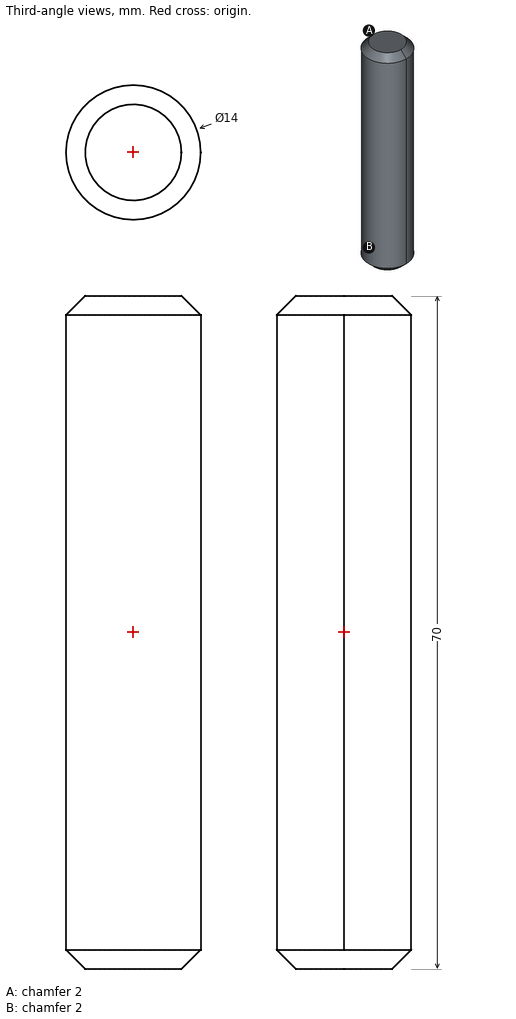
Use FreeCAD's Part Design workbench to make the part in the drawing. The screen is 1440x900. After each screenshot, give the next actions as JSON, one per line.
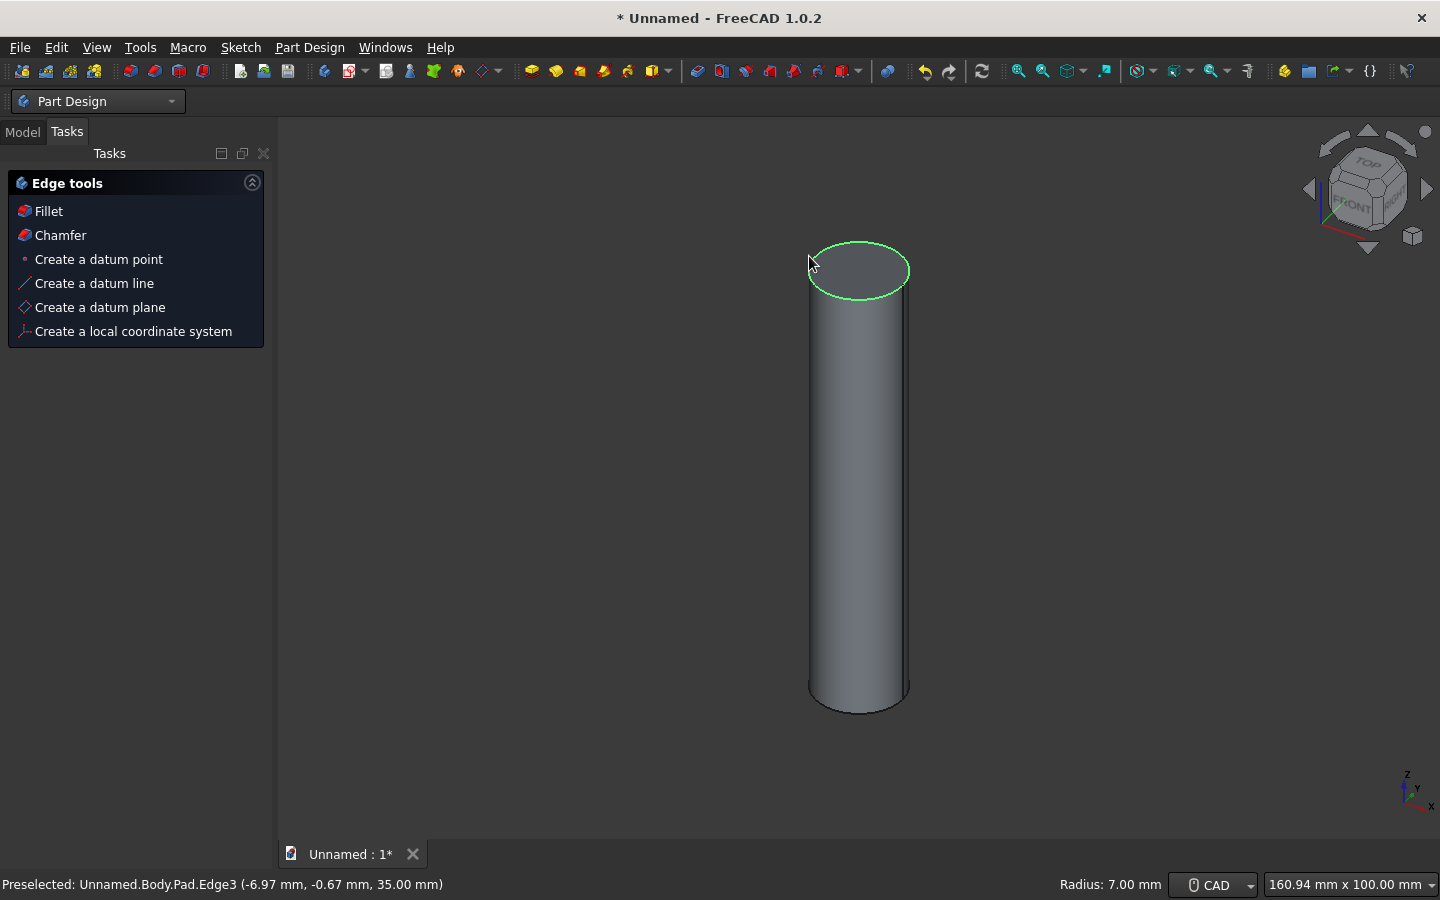
{"action": "left_click", "coordinate": [156, 72]}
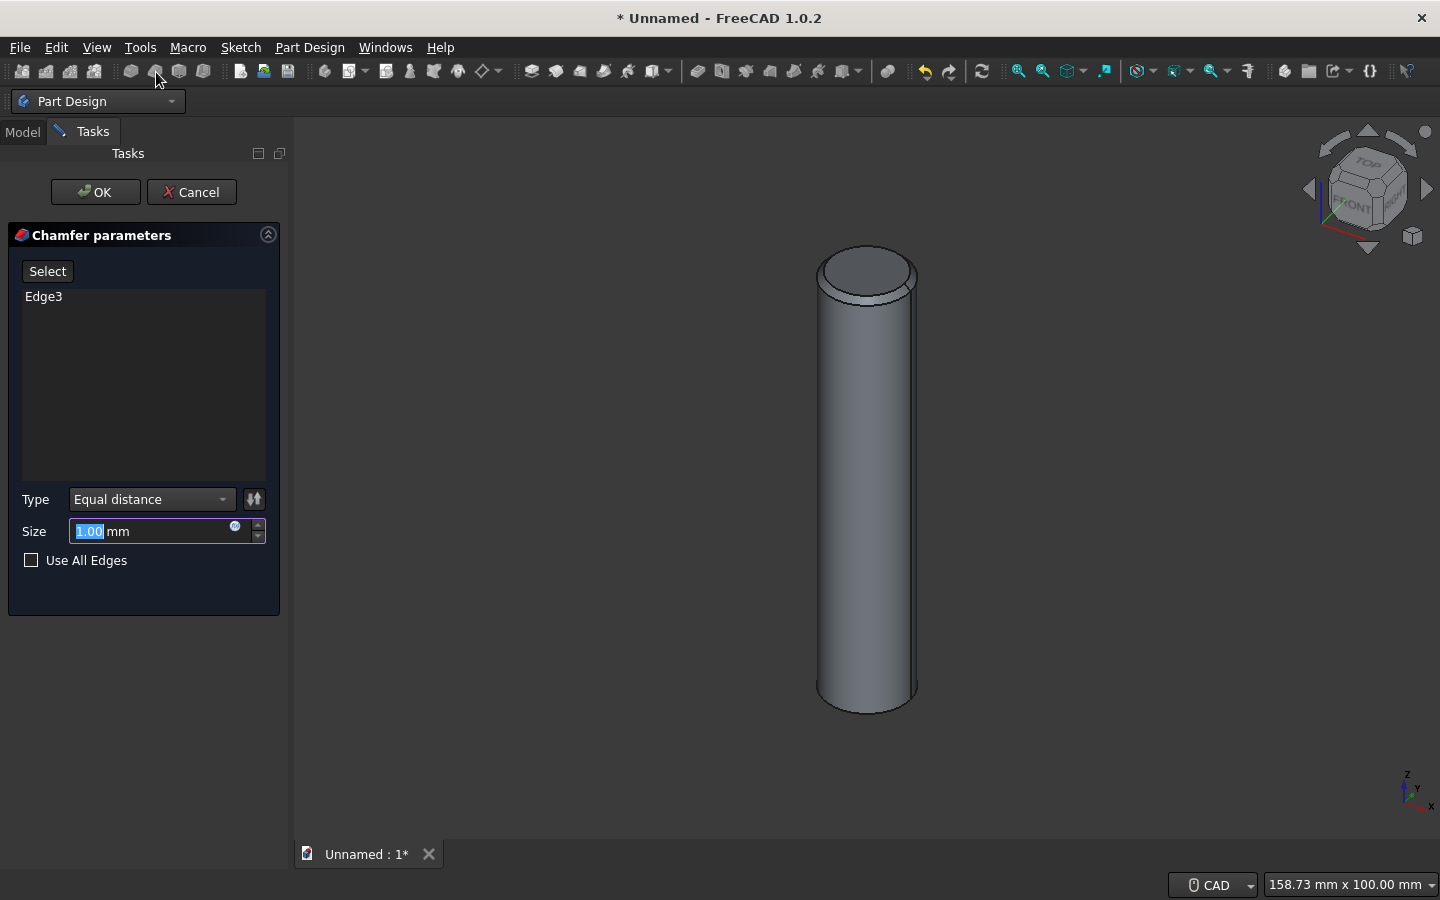
{"action": "type", "text": "2"}
{"action": "key", "text": "Tab"}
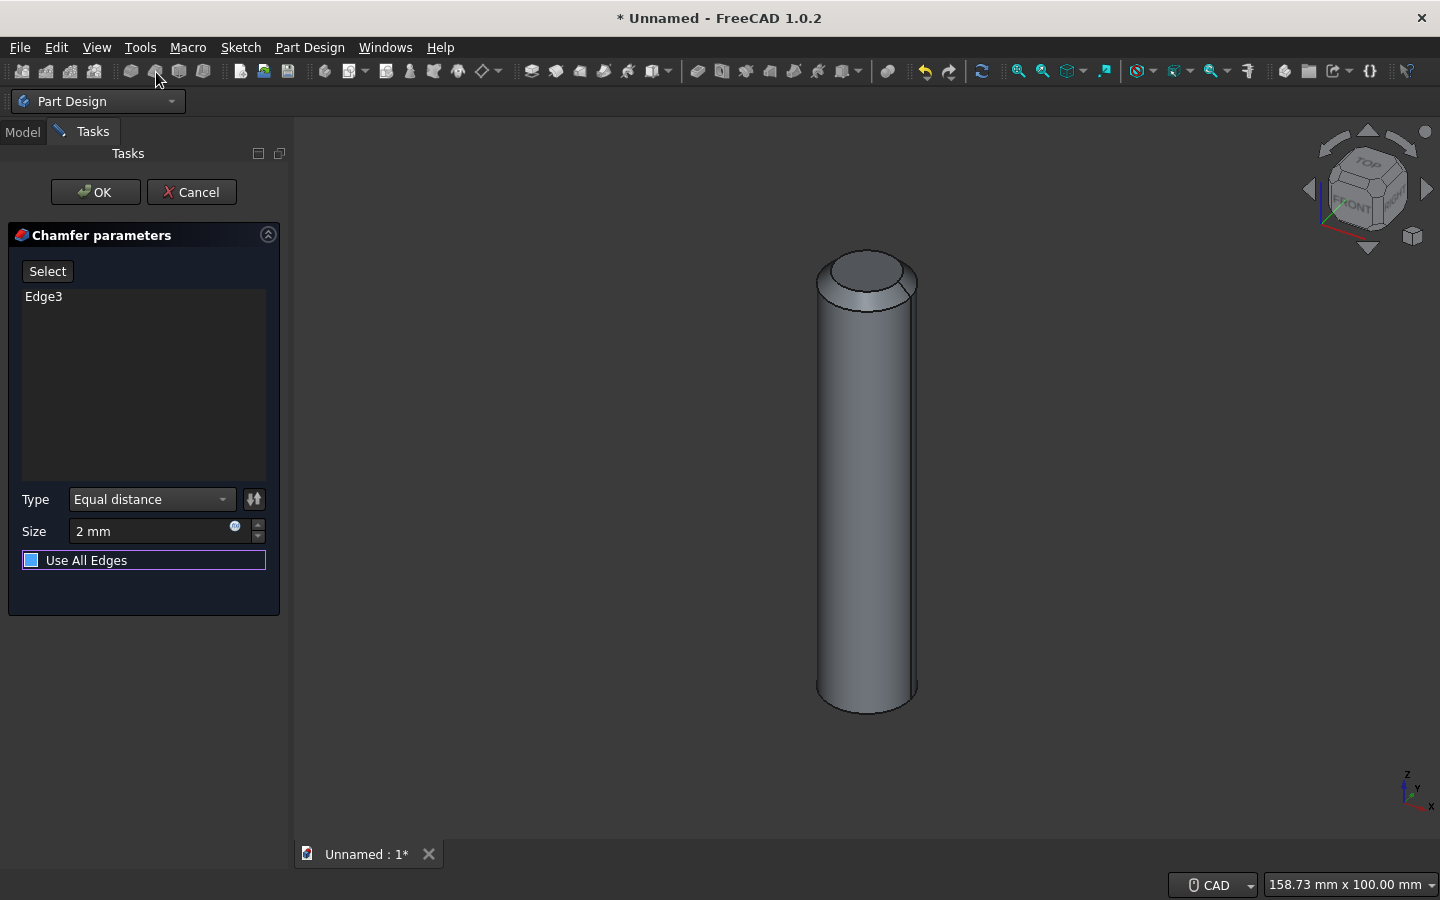
{"action": "left_click", "coordinate": [96, 192]}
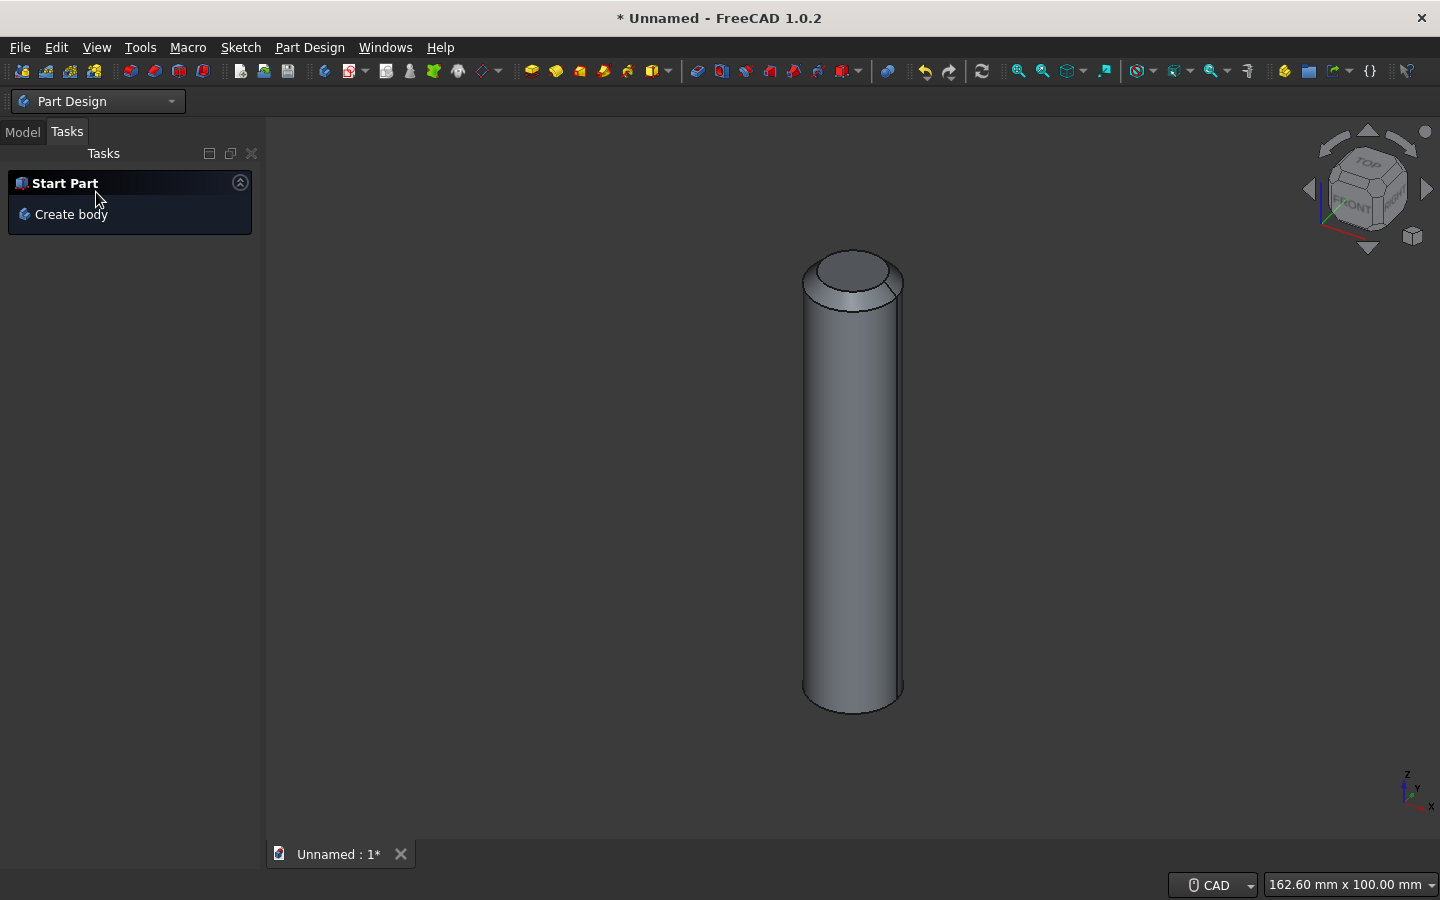
{"action": "key", "text": "0"}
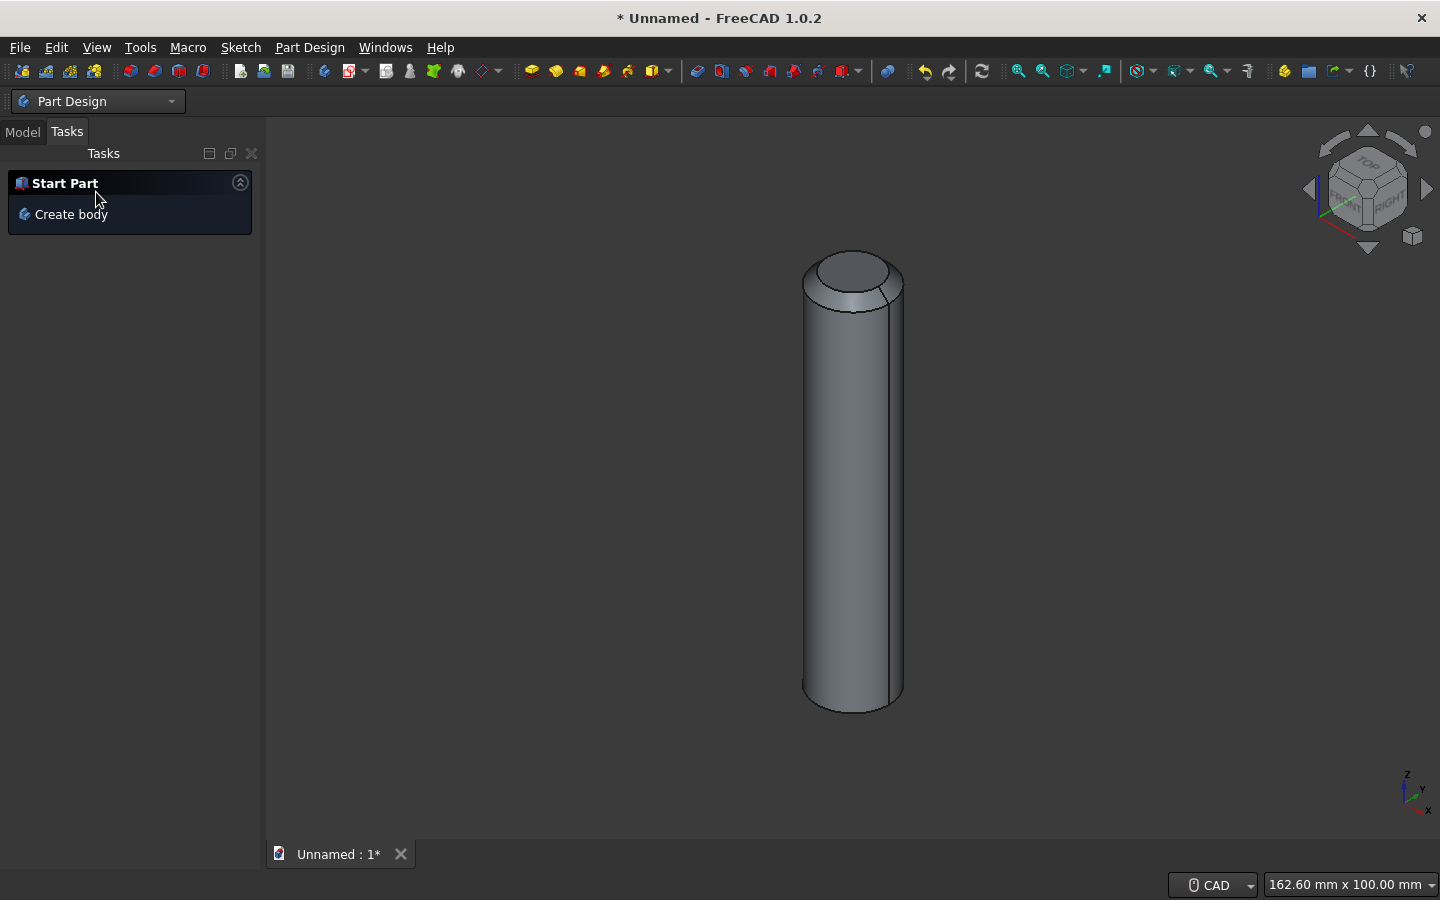
{"action": "key", "text": "2"}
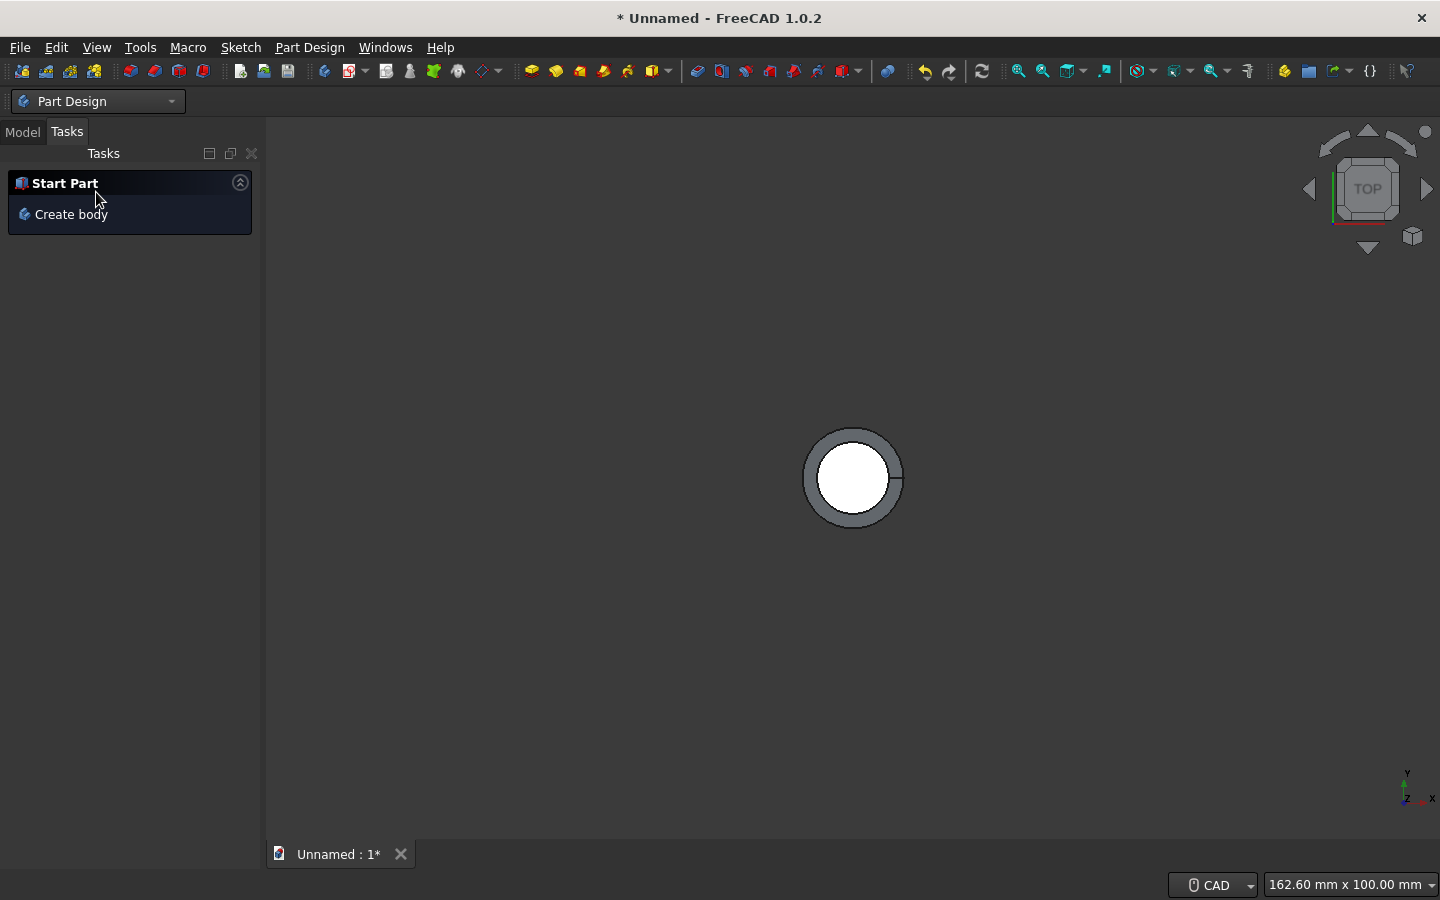
{"action": "key", "text": "v f"}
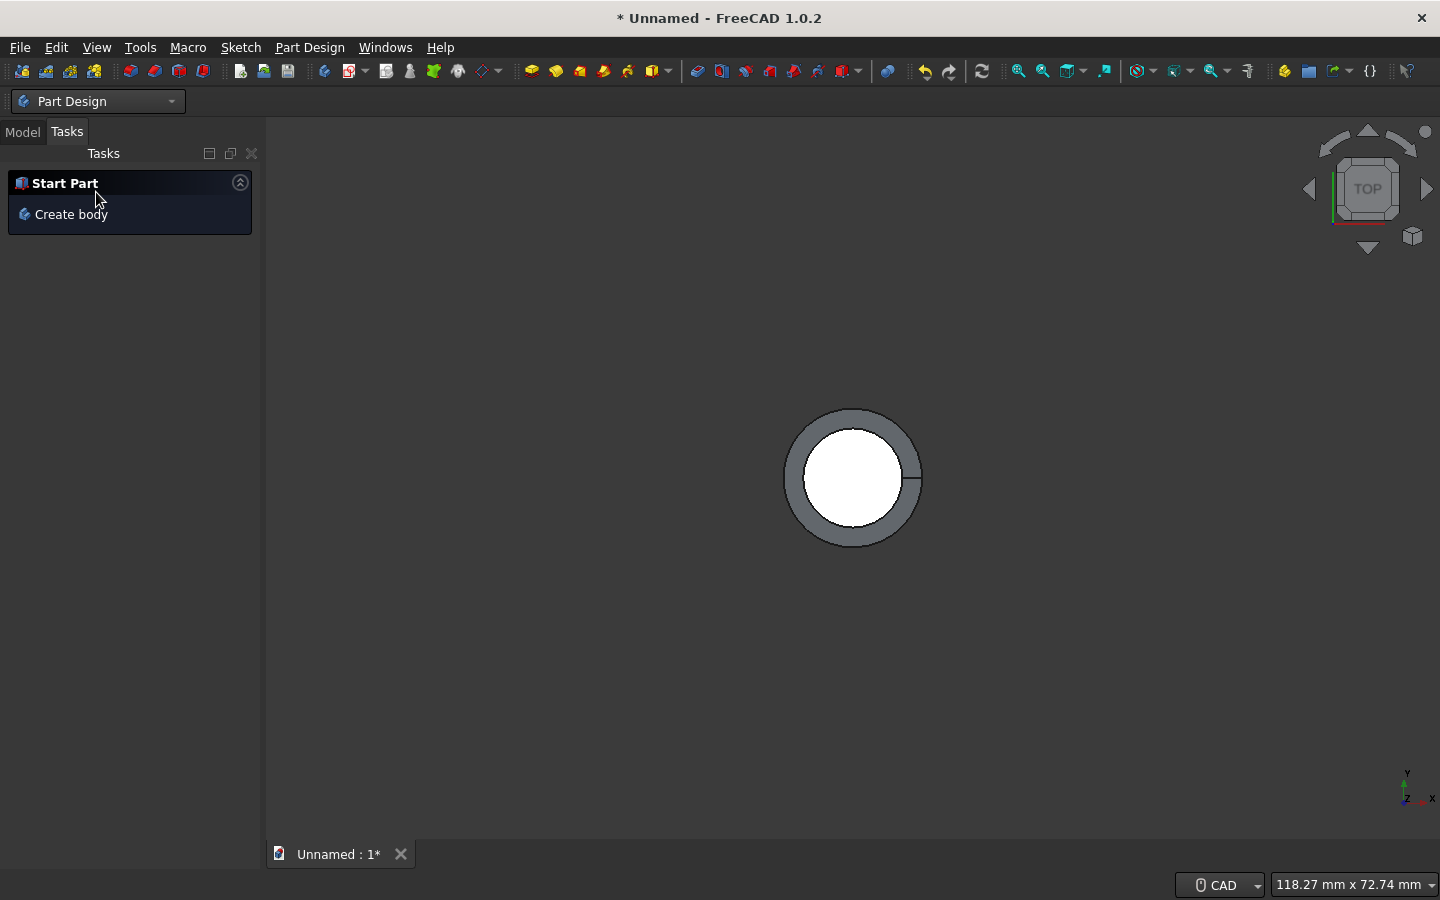
{"action": "key", "text": "1"}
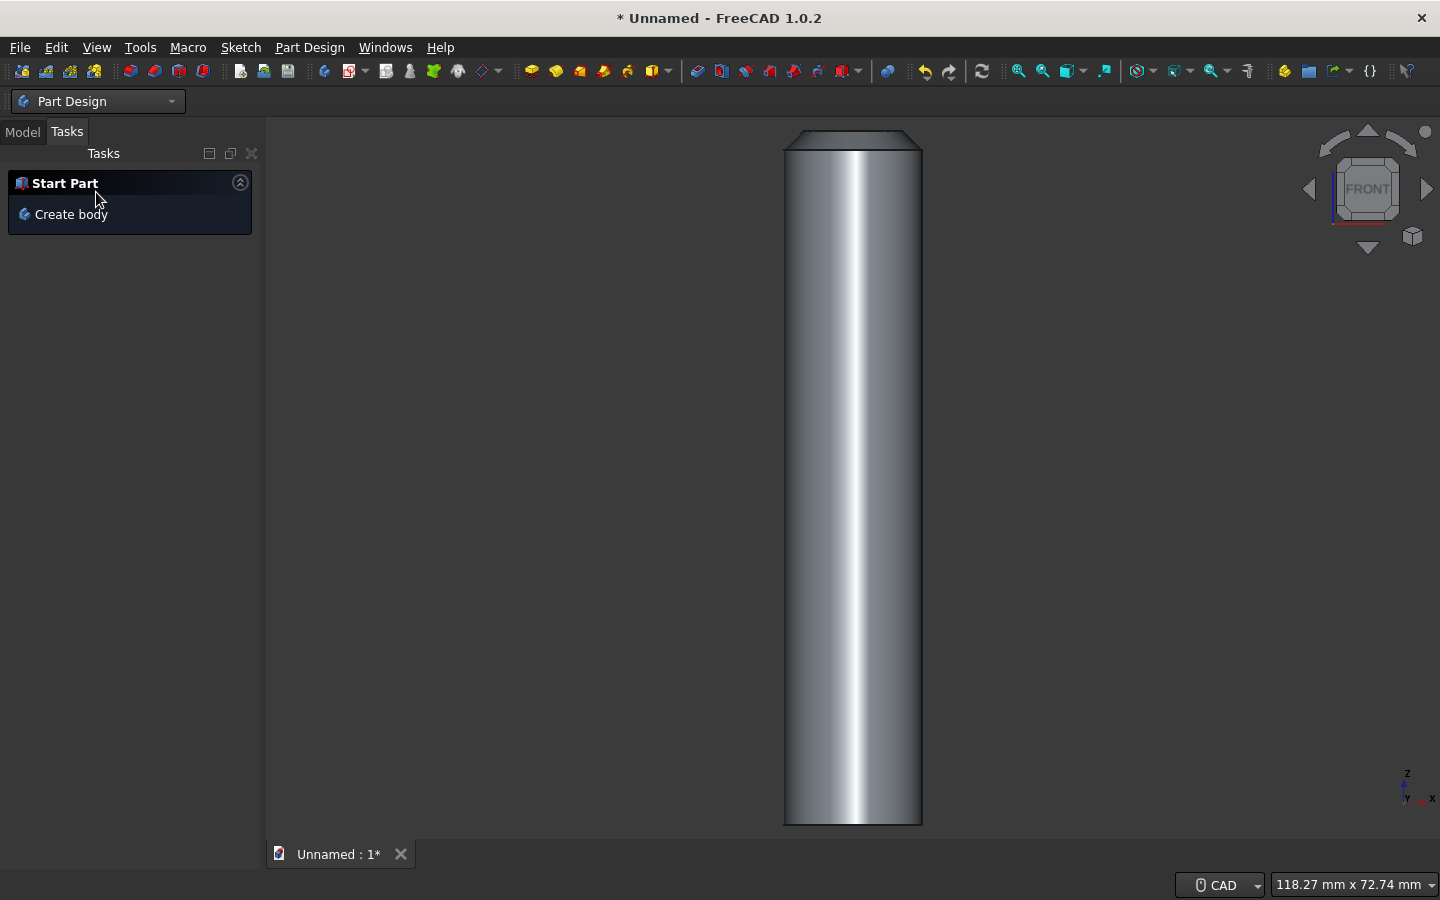
{"action": "key", "text": "3"}